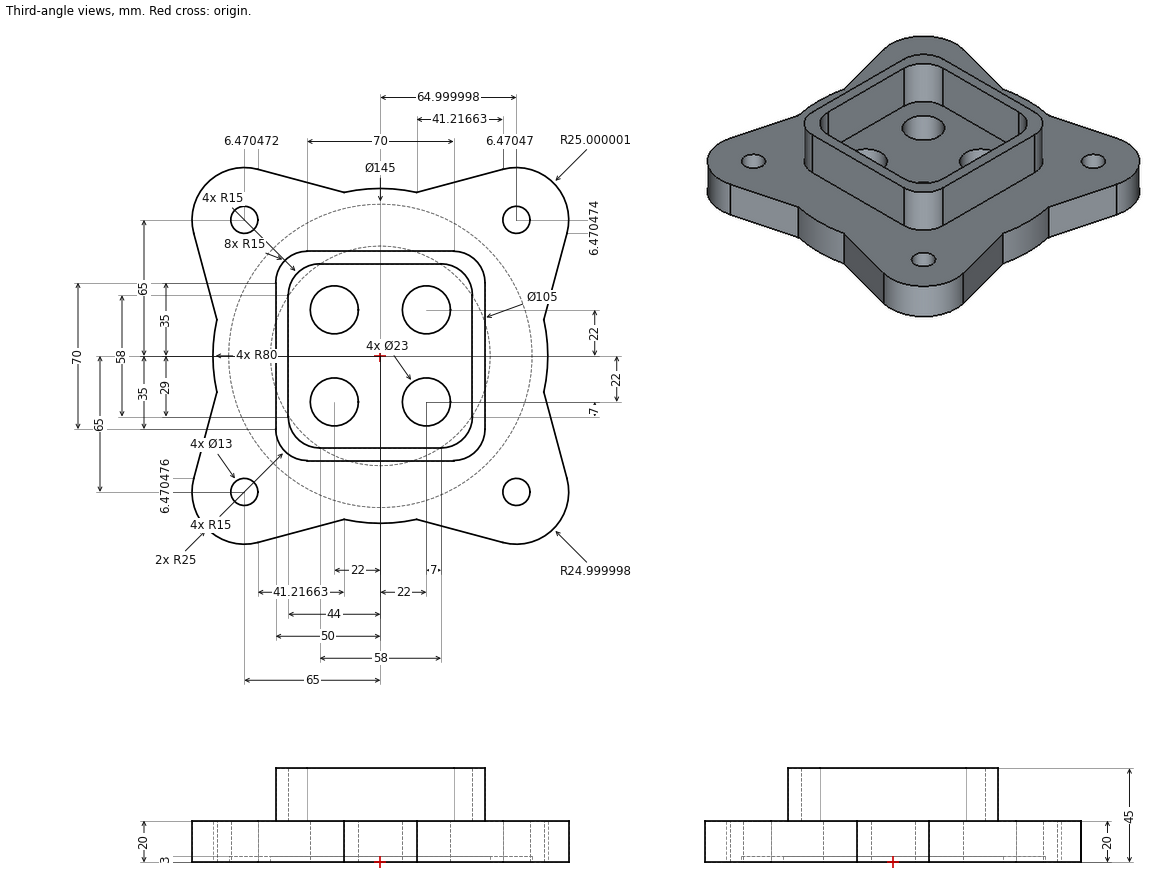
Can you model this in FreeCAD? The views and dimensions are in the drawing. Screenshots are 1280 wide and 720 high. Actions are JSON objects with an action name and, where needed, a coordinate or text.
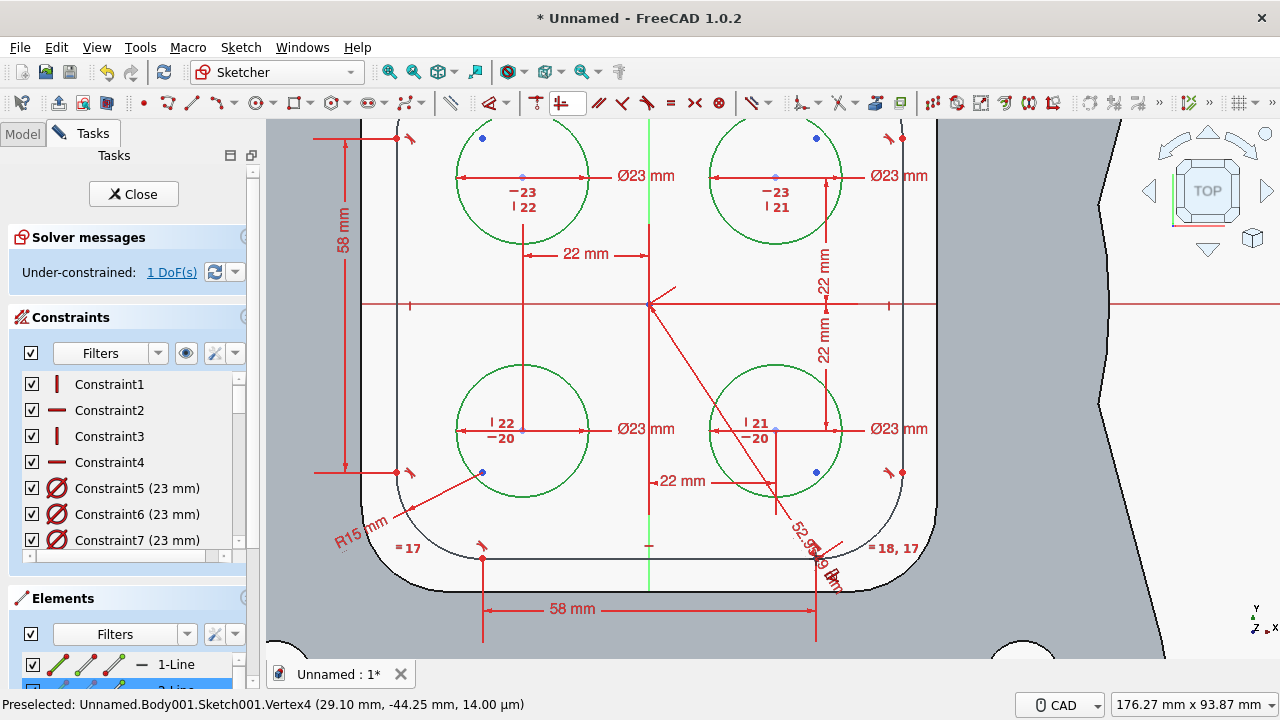
{"action": "left_click", "coordinate": [776, 431]}
{"action": "left_click", "coordinate": [796, 593]}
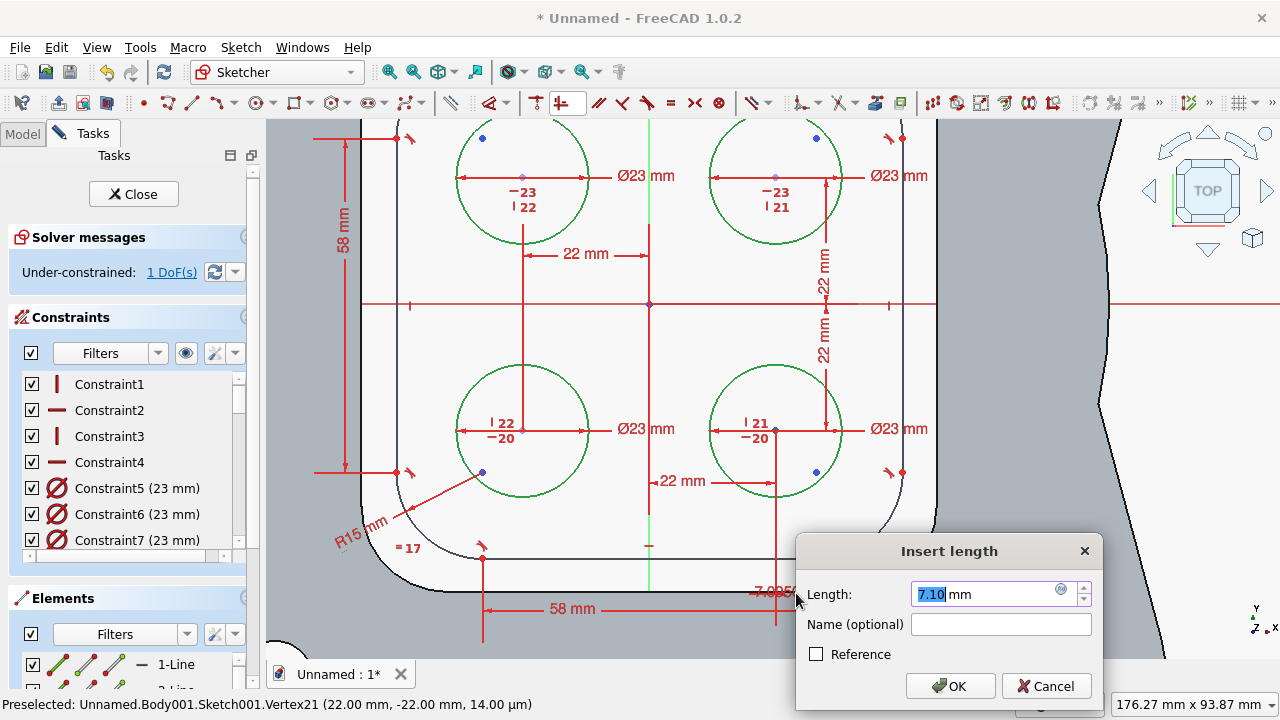
{"action": "type", "text": "7"}
{"action": "key", "text": "Return"}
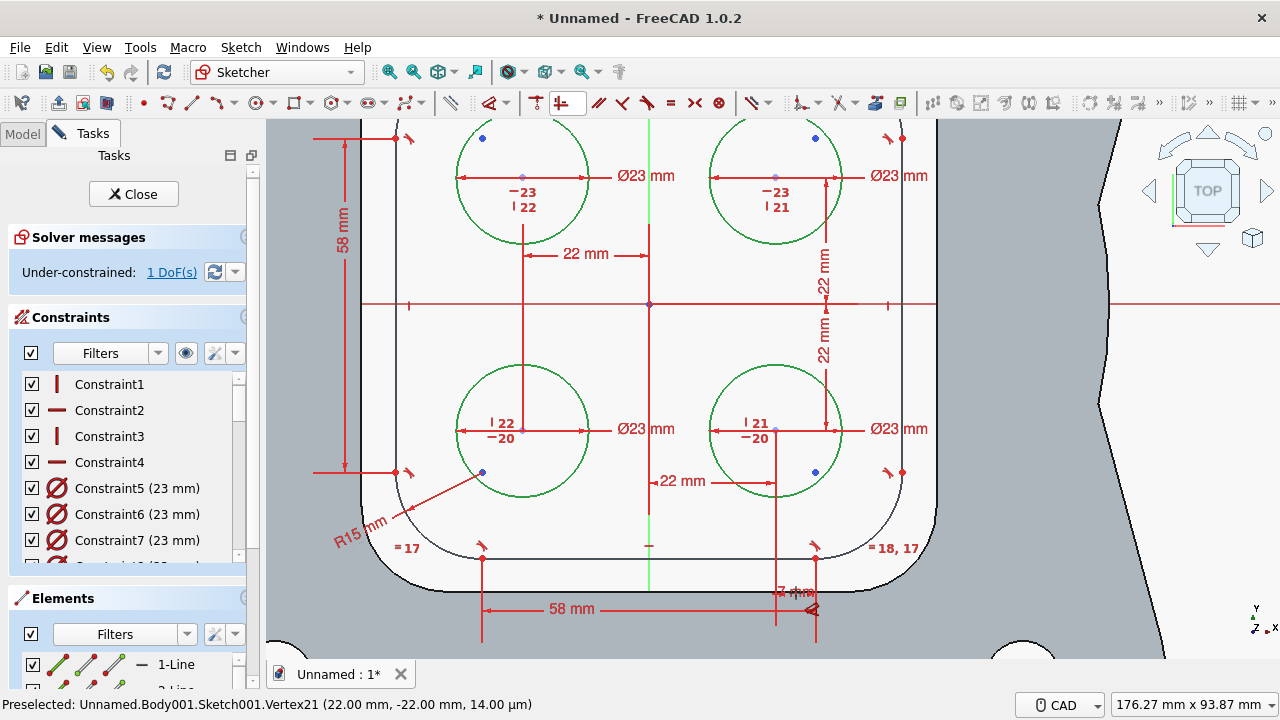
{"action": "left_click", "coordinate": [902, 473]}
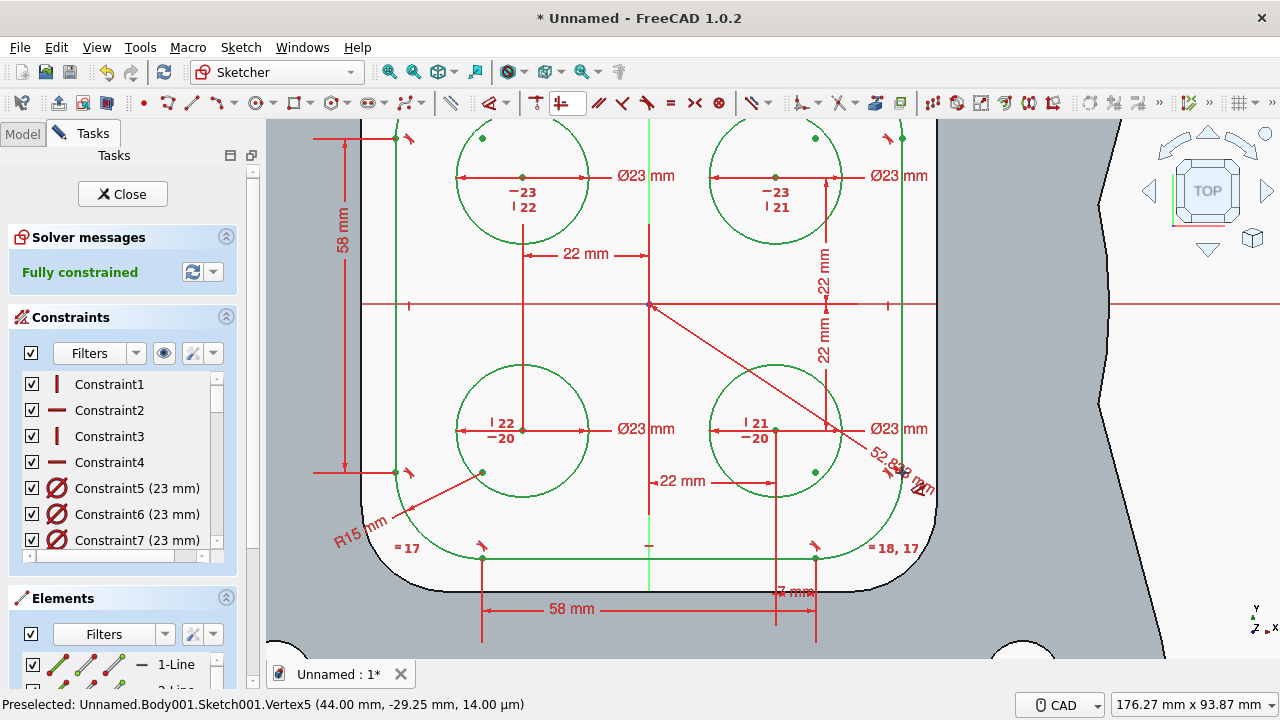
{"action": "left_click", "coordinate": [776, 431]}
{"action": "left_click", "coordinate": [936, 452]}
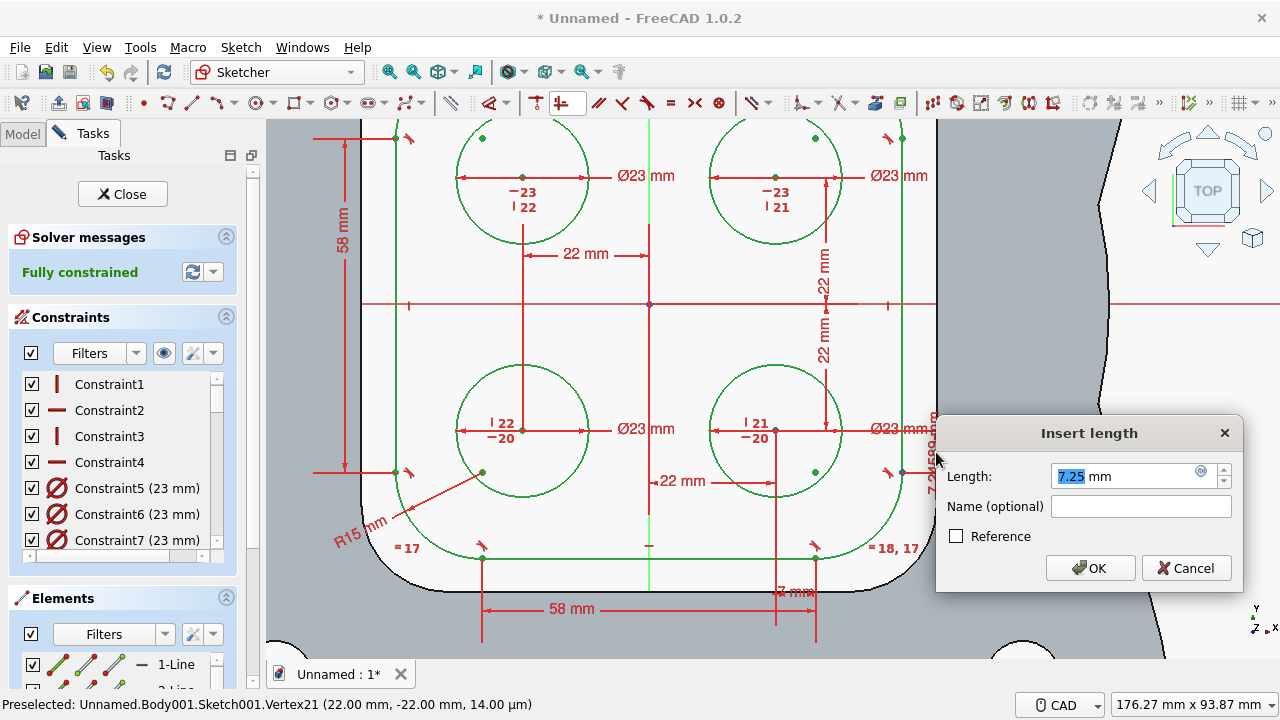
{"action": "type", "text": "7"}
{"action": "key", "text": "Return"}
{"action": "key", "text": "Escape"}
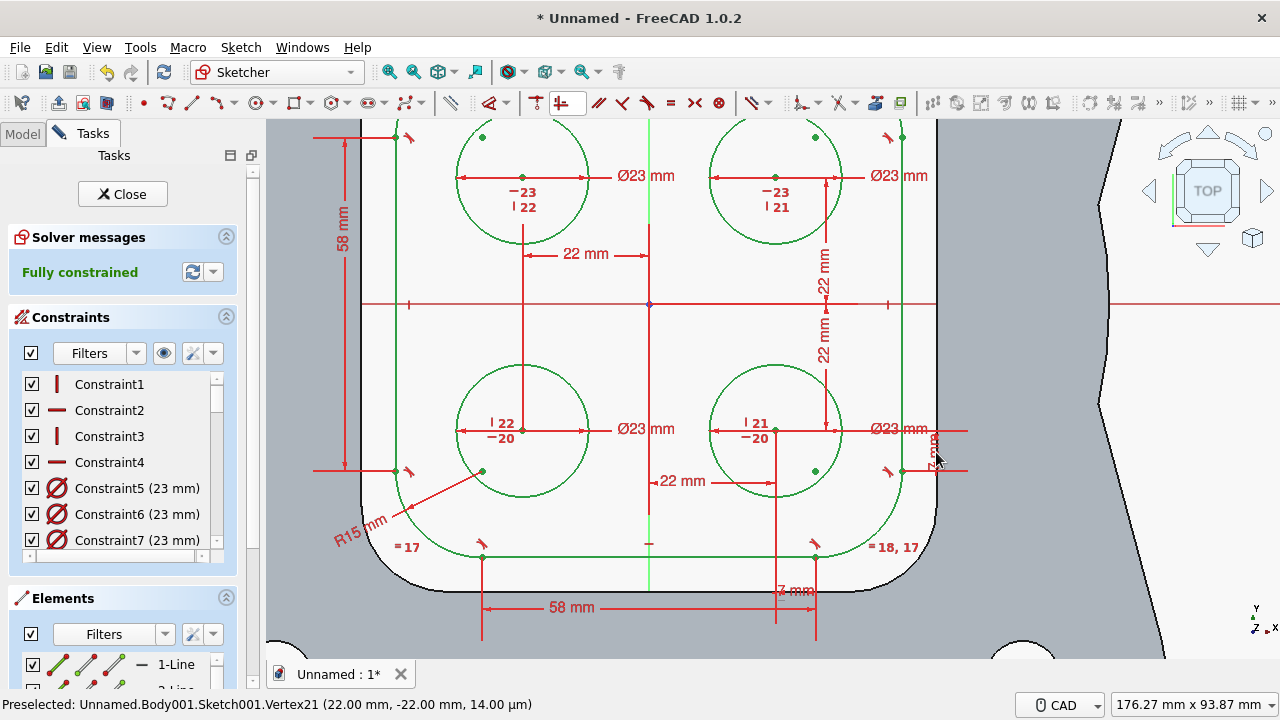
{"action": "left_click", "coordinate": [123, 194]}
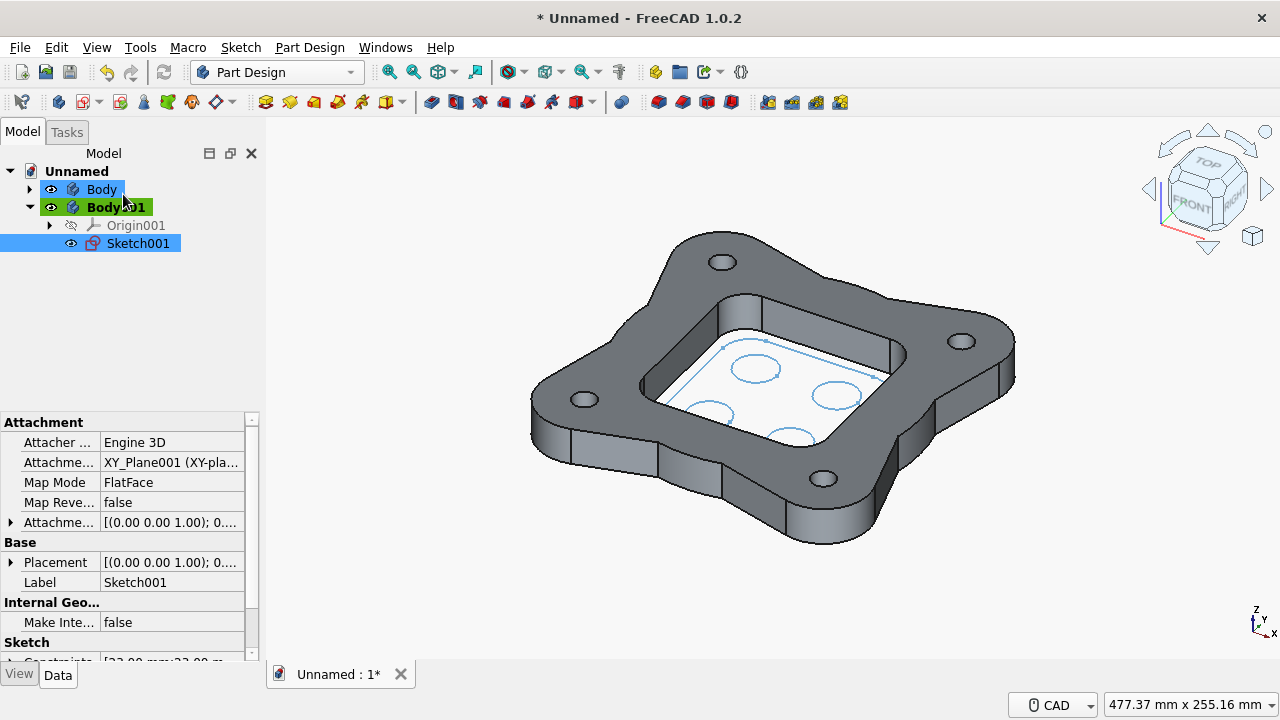
{"action": "left_click", "coordinate": [266, 102]}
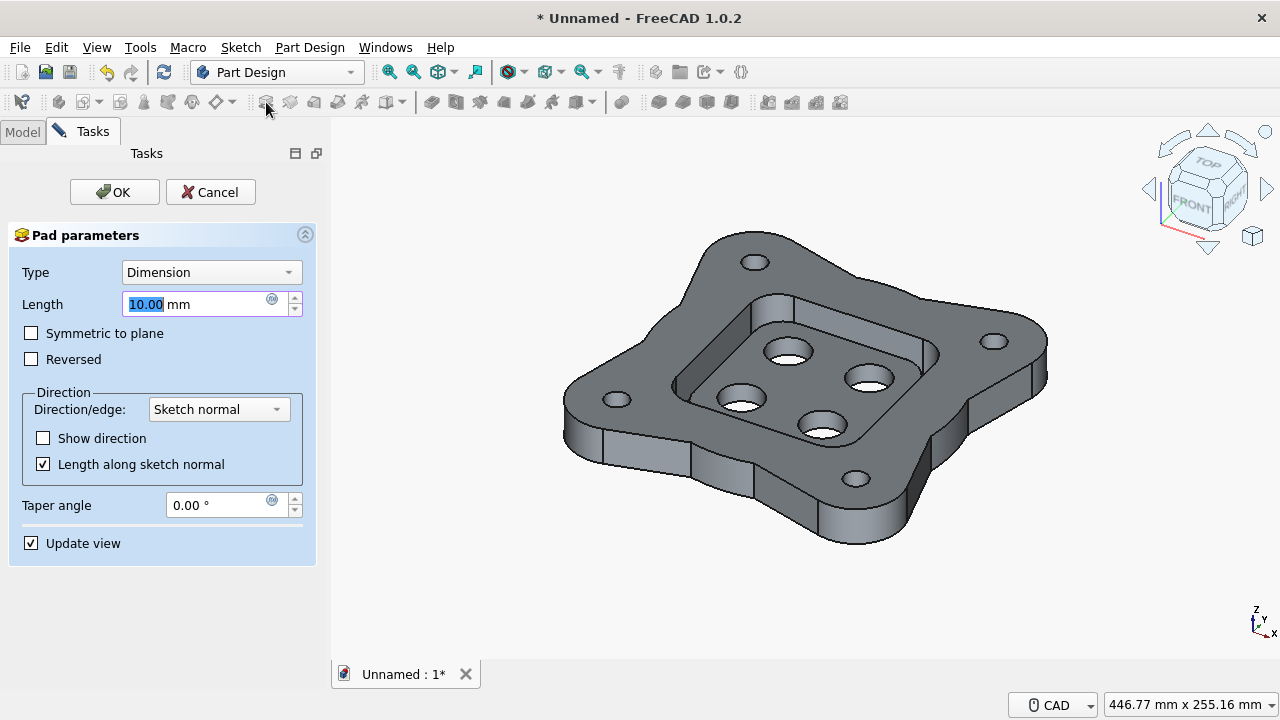
{"action": "type", "text": "20"}
{"action": "key", "text": "Tab"}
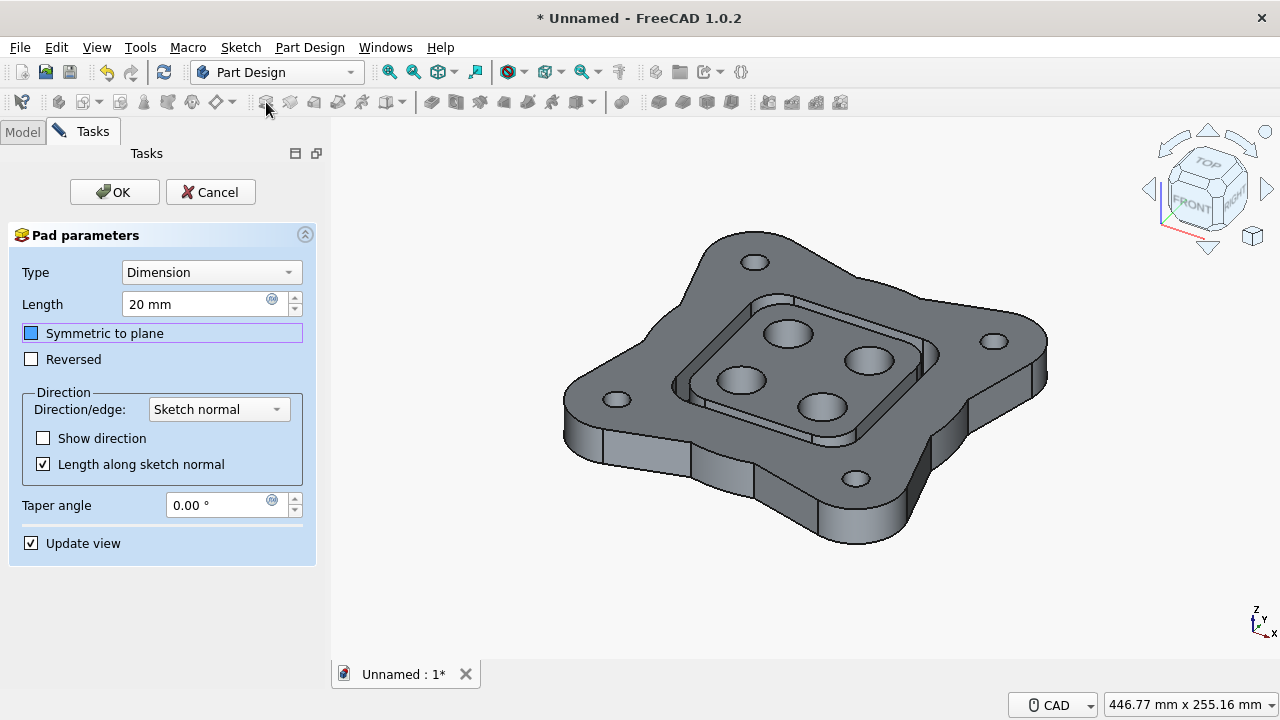
{"action": "left_click", "coordinate": [115, 192]}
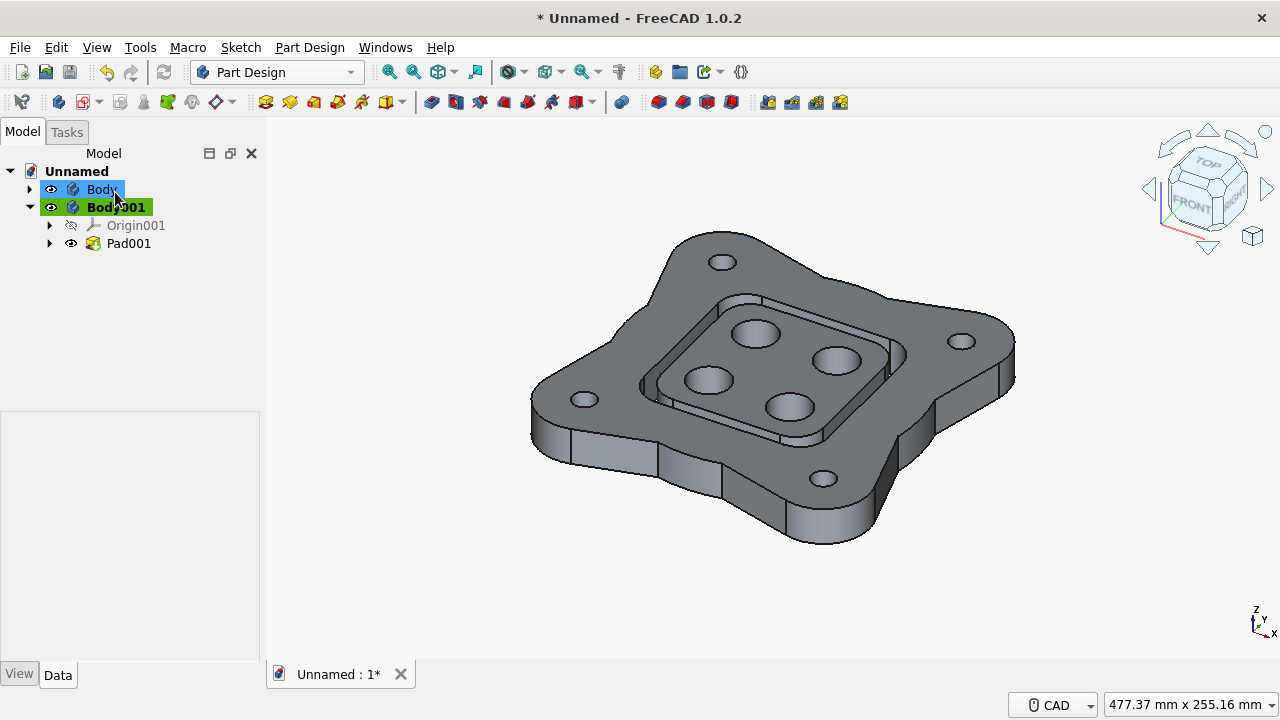
{"action": "left_click", "coordinate": [390, 72]}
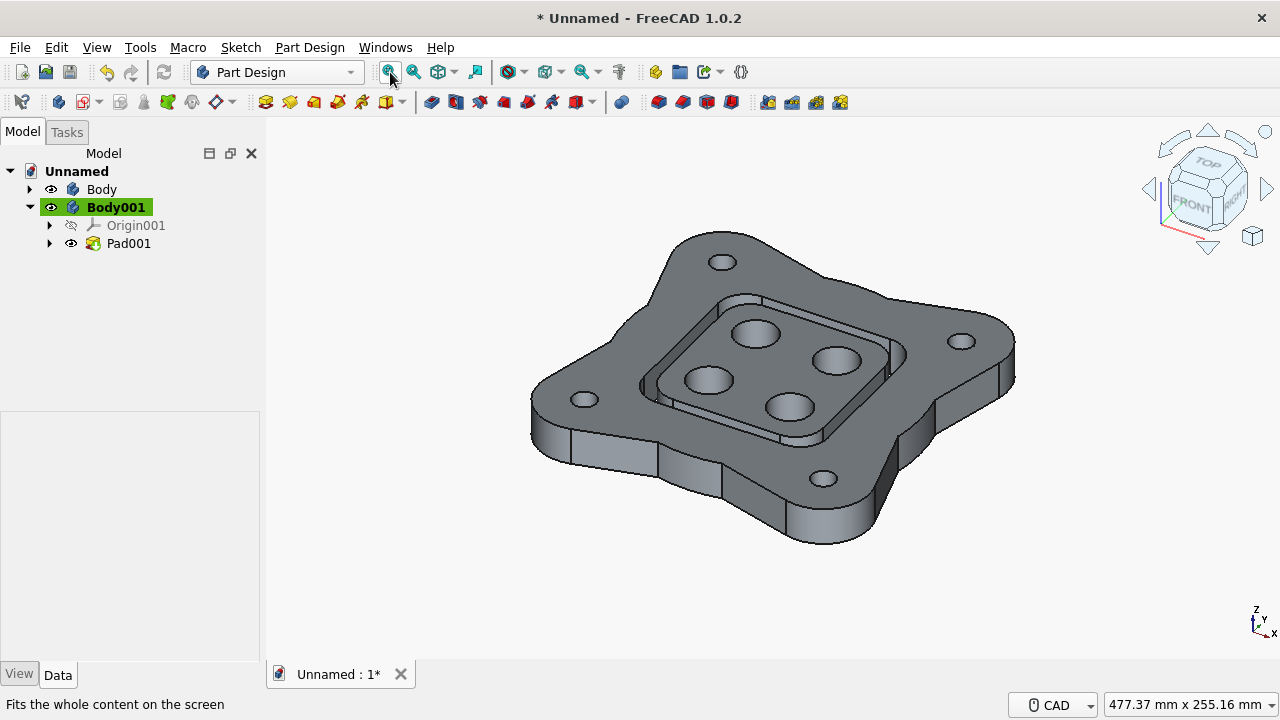
{"action": "double_click", "coordinate": [96, 189]}